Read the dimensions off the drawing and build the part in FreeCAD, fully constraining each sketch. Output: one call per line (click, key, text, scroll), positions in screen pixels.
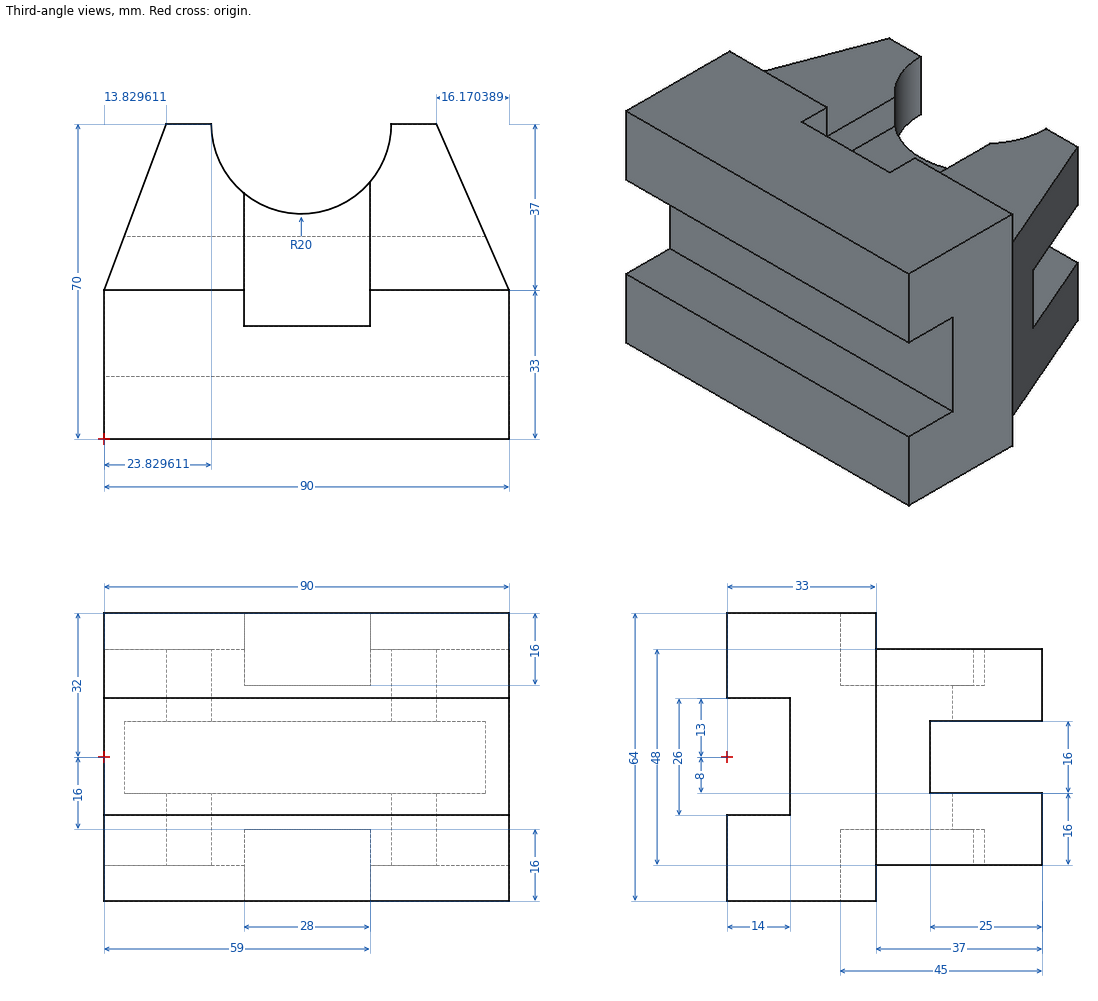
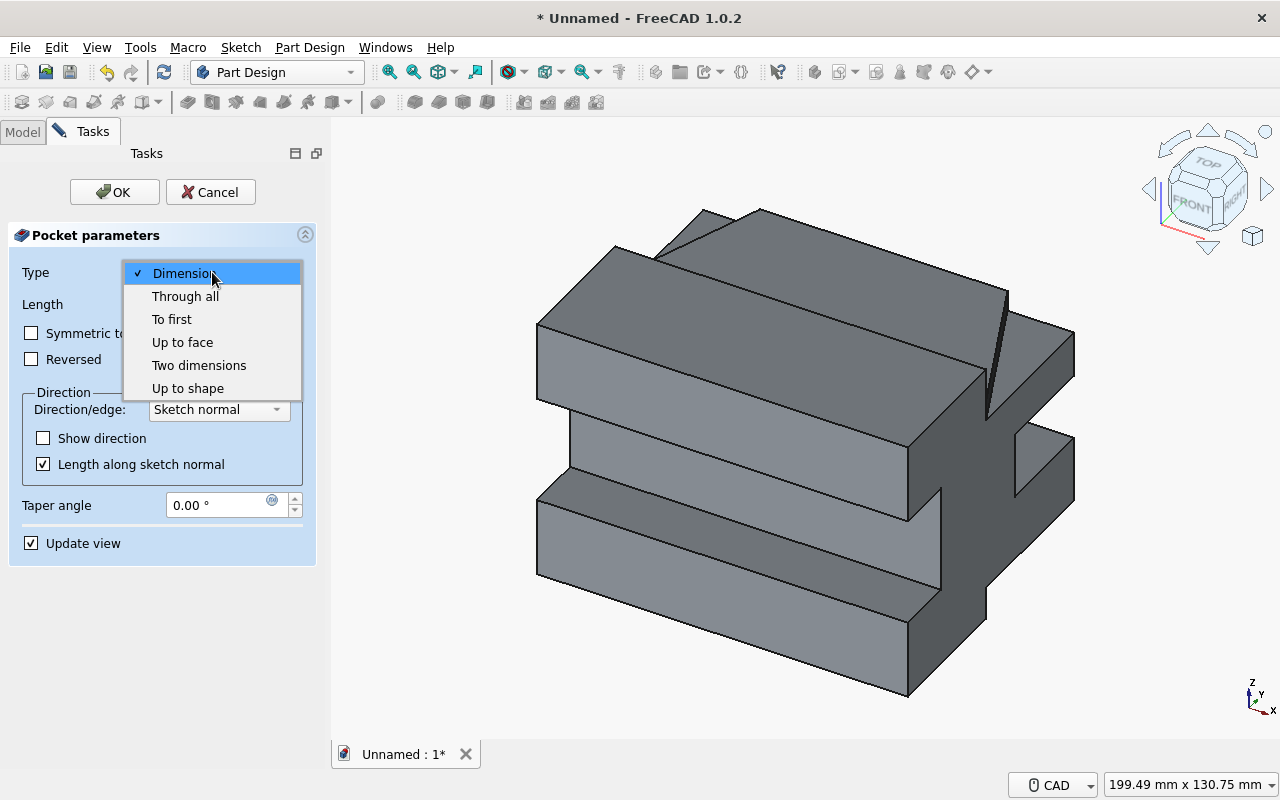
click(212, 296)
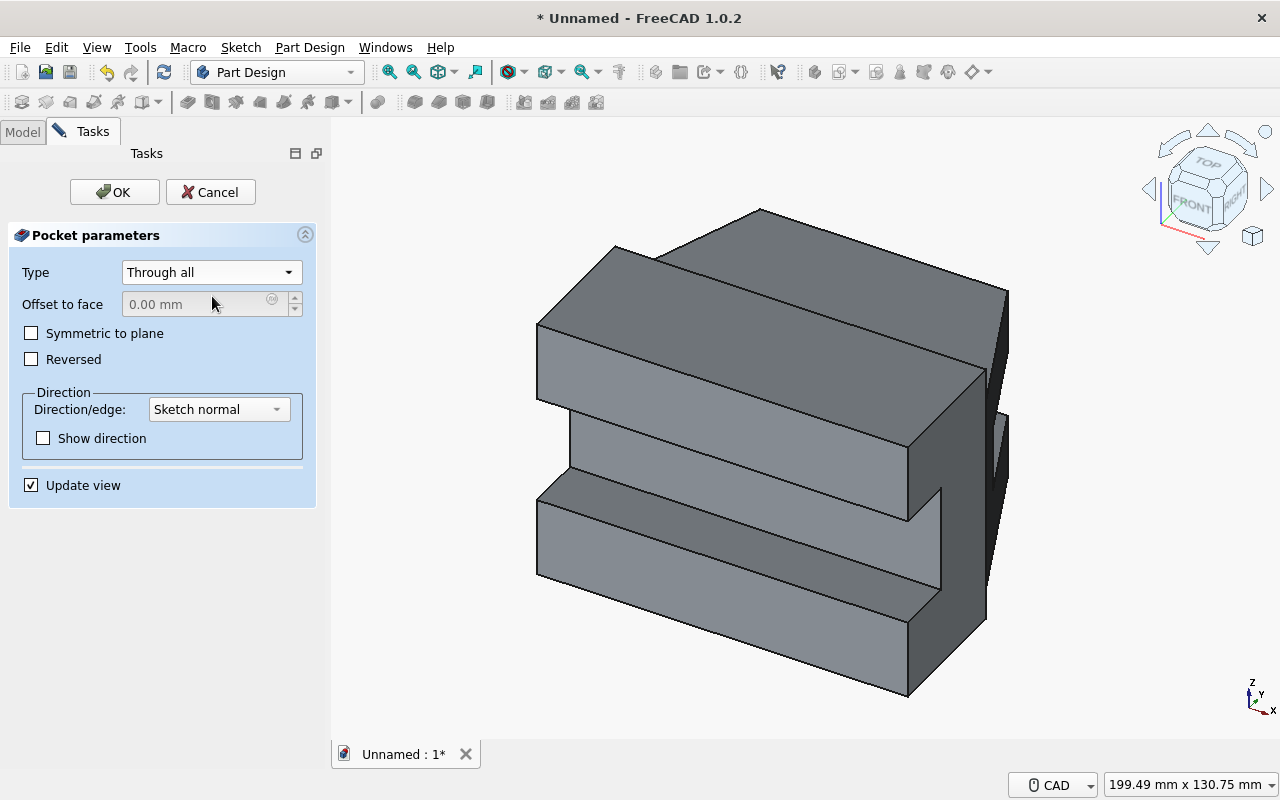
click(115, 192)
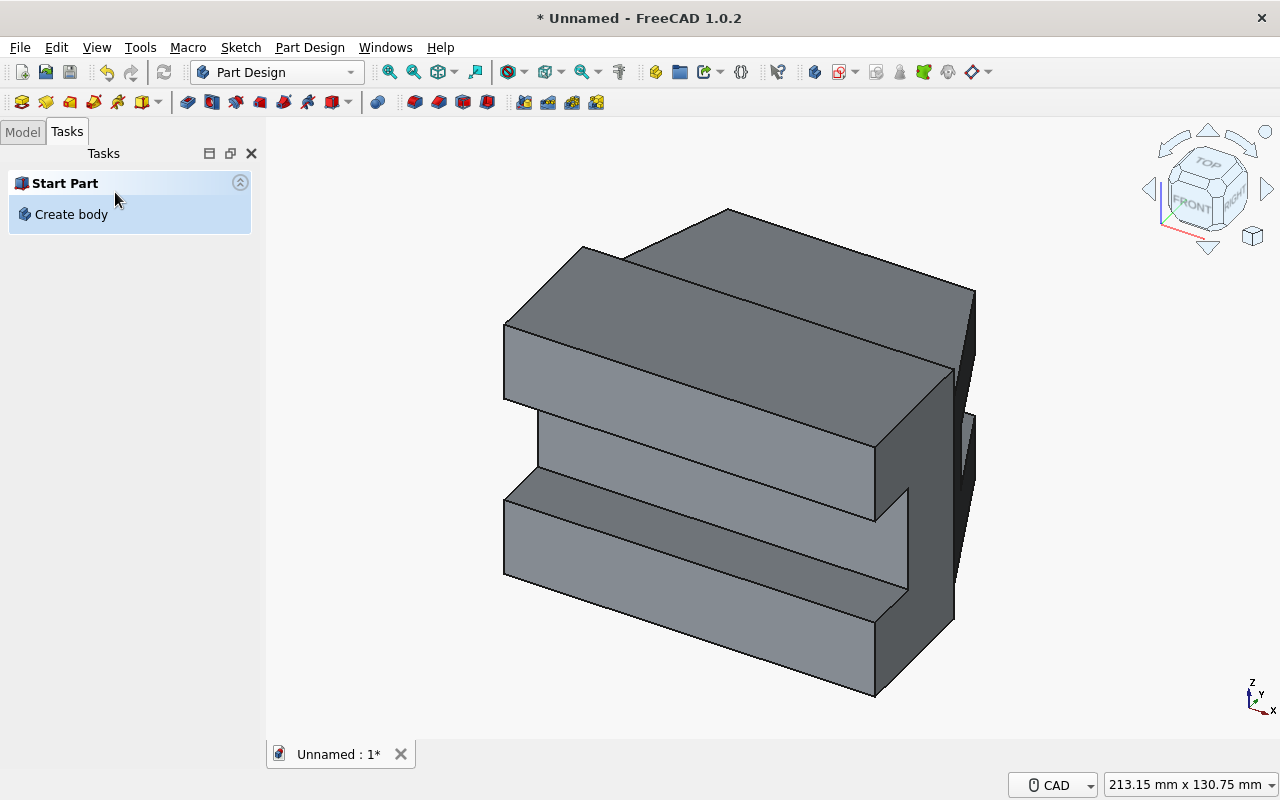
key(5)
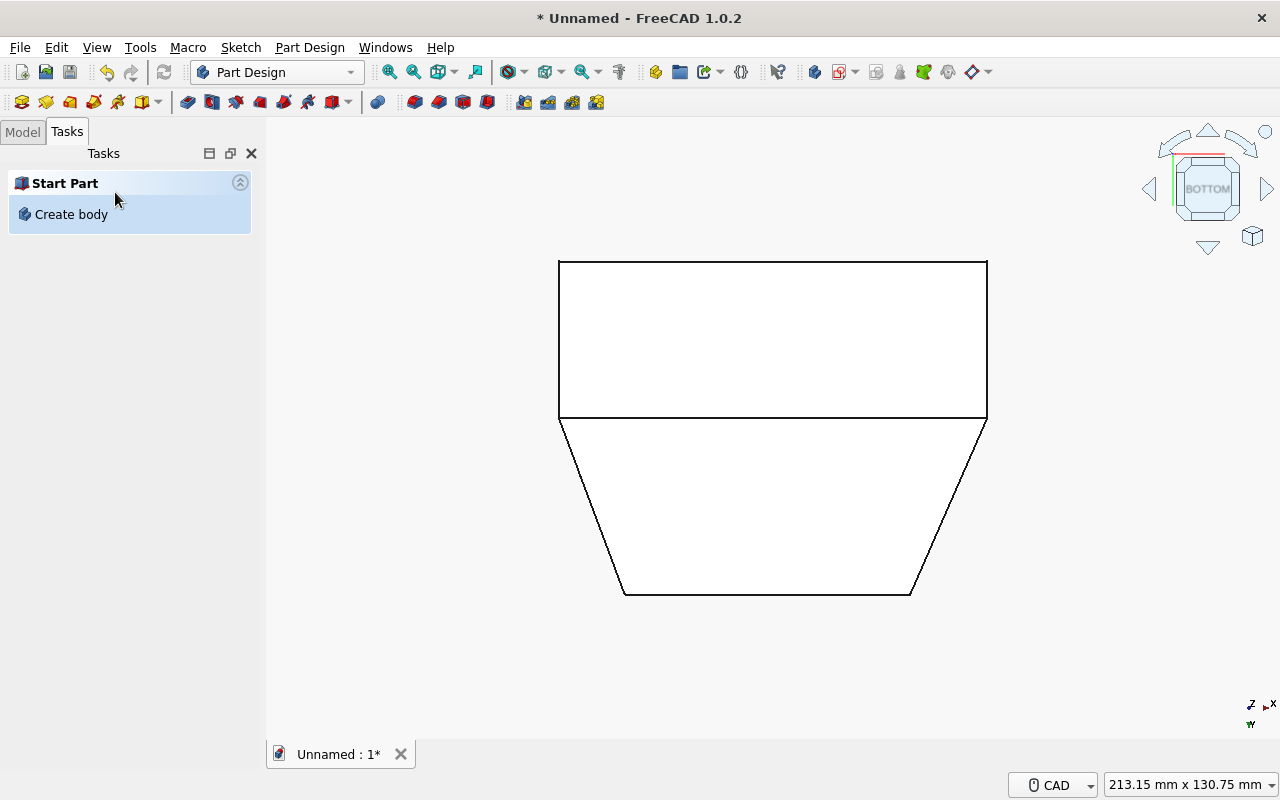
click(834, 505)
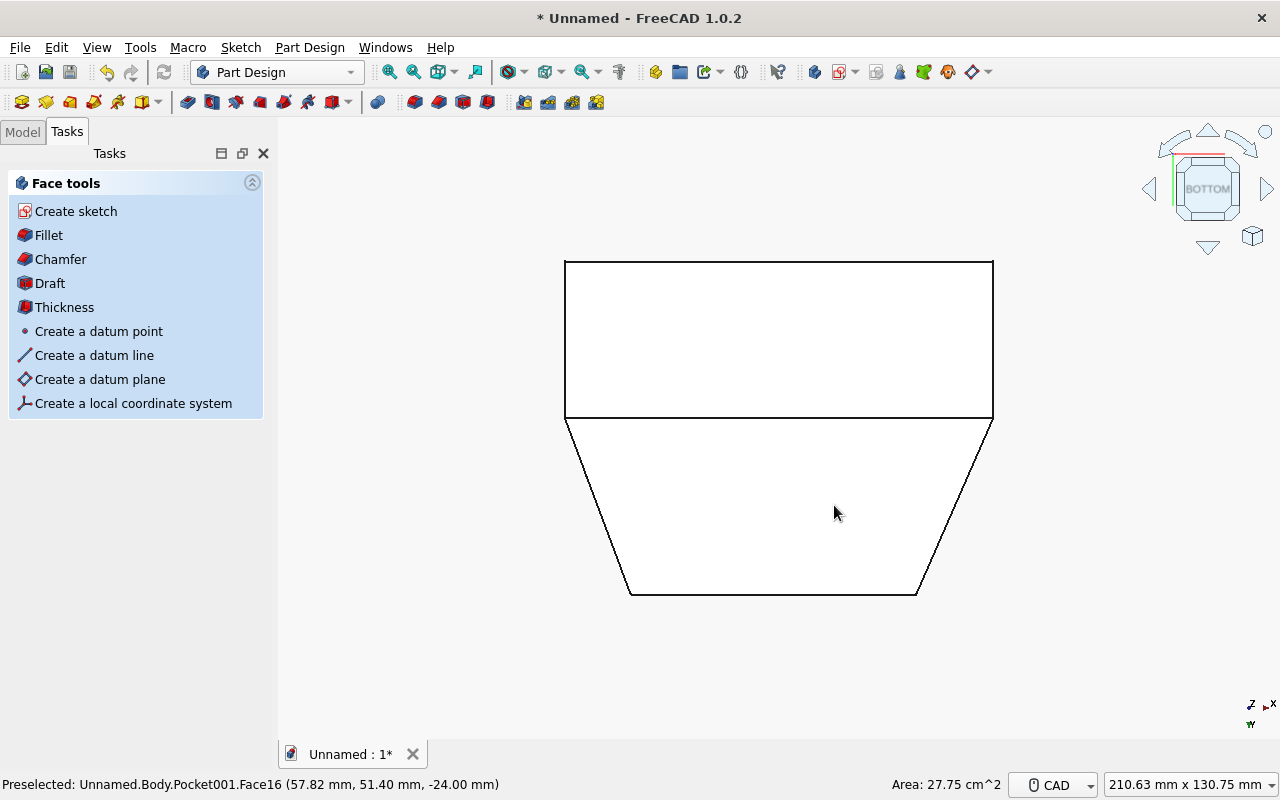
click(840, 72)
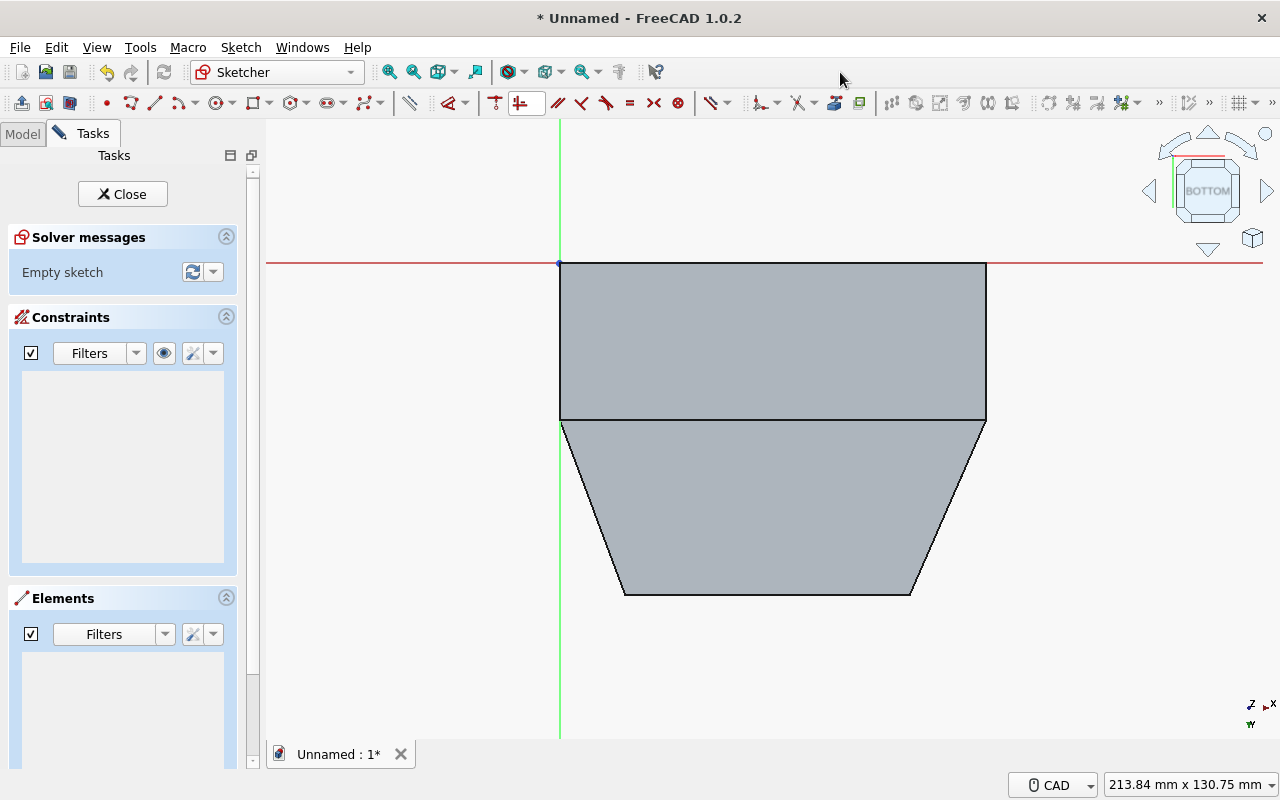
click(156, 104)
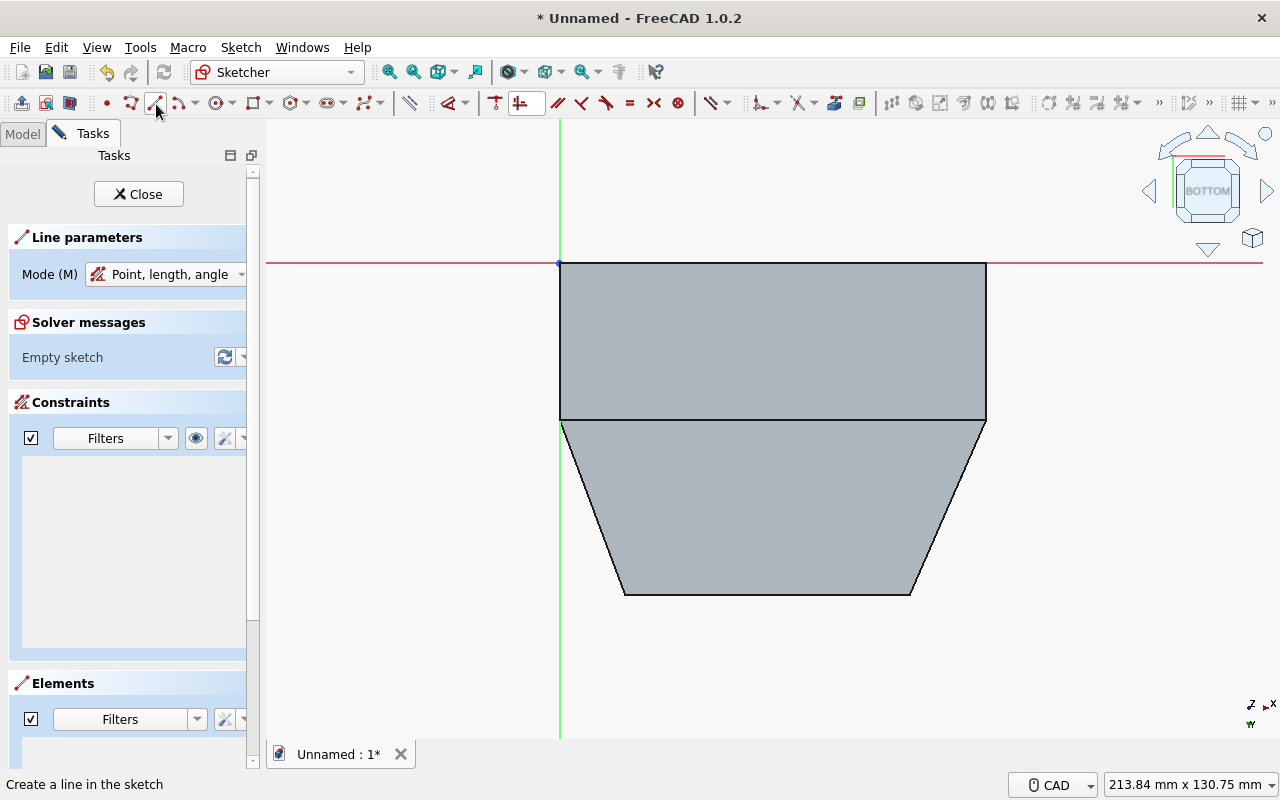
click(673, 595)
click(862, 595)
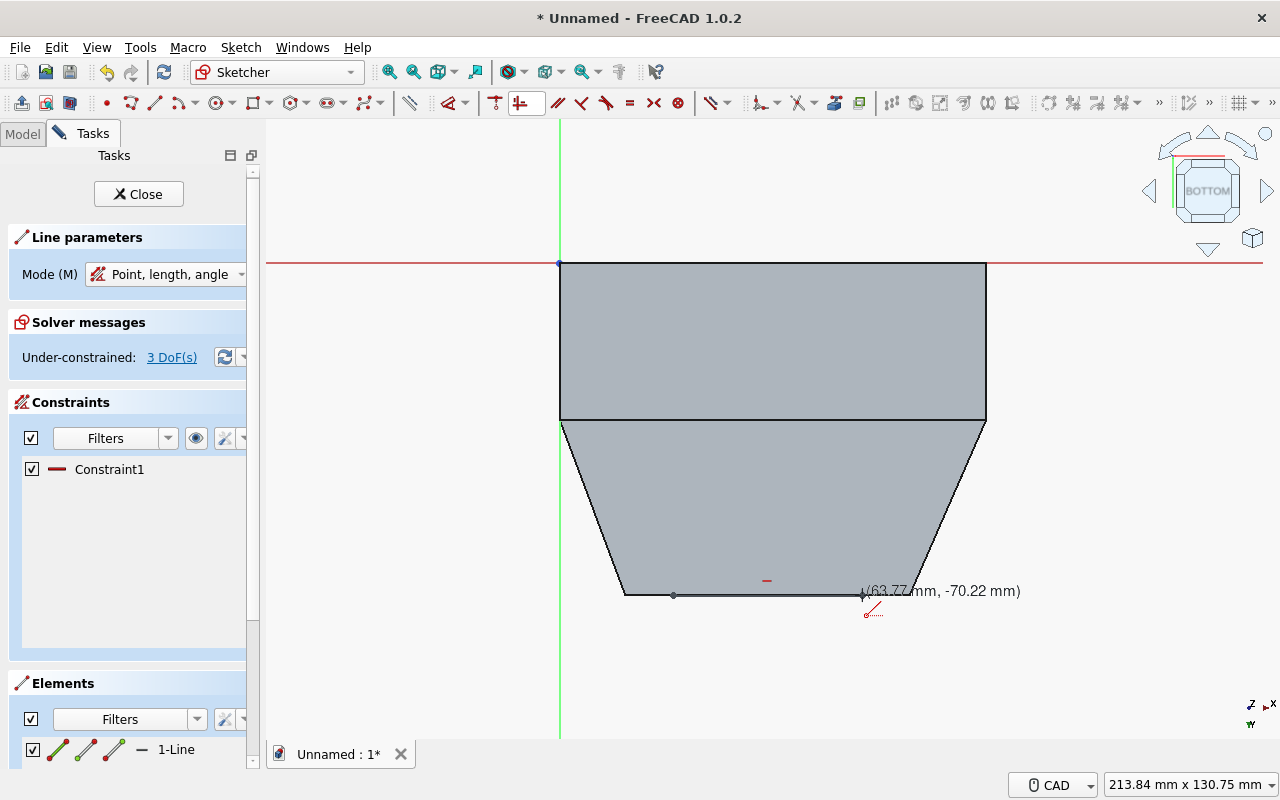
key(g)
key(3)
key(a)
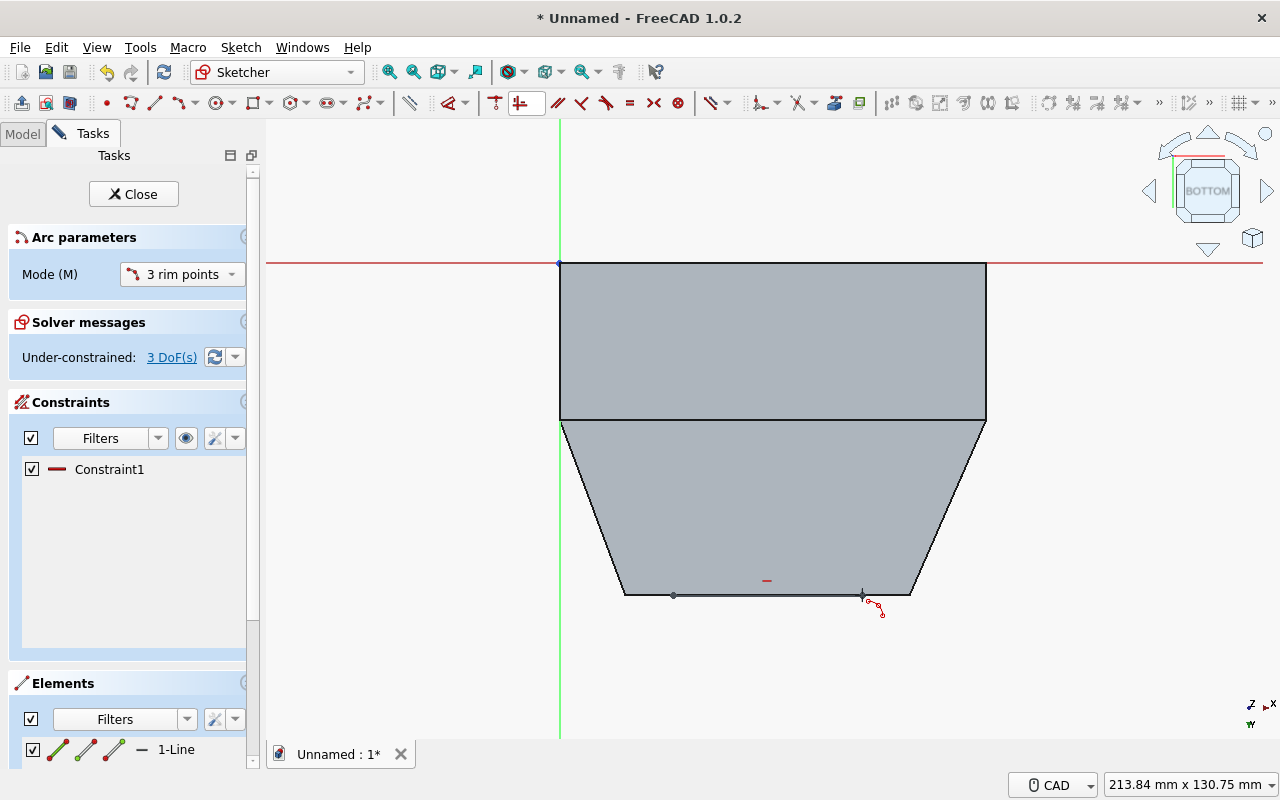
click(862, 596)
click(673, 596)
click(767, 500)
key(Escape)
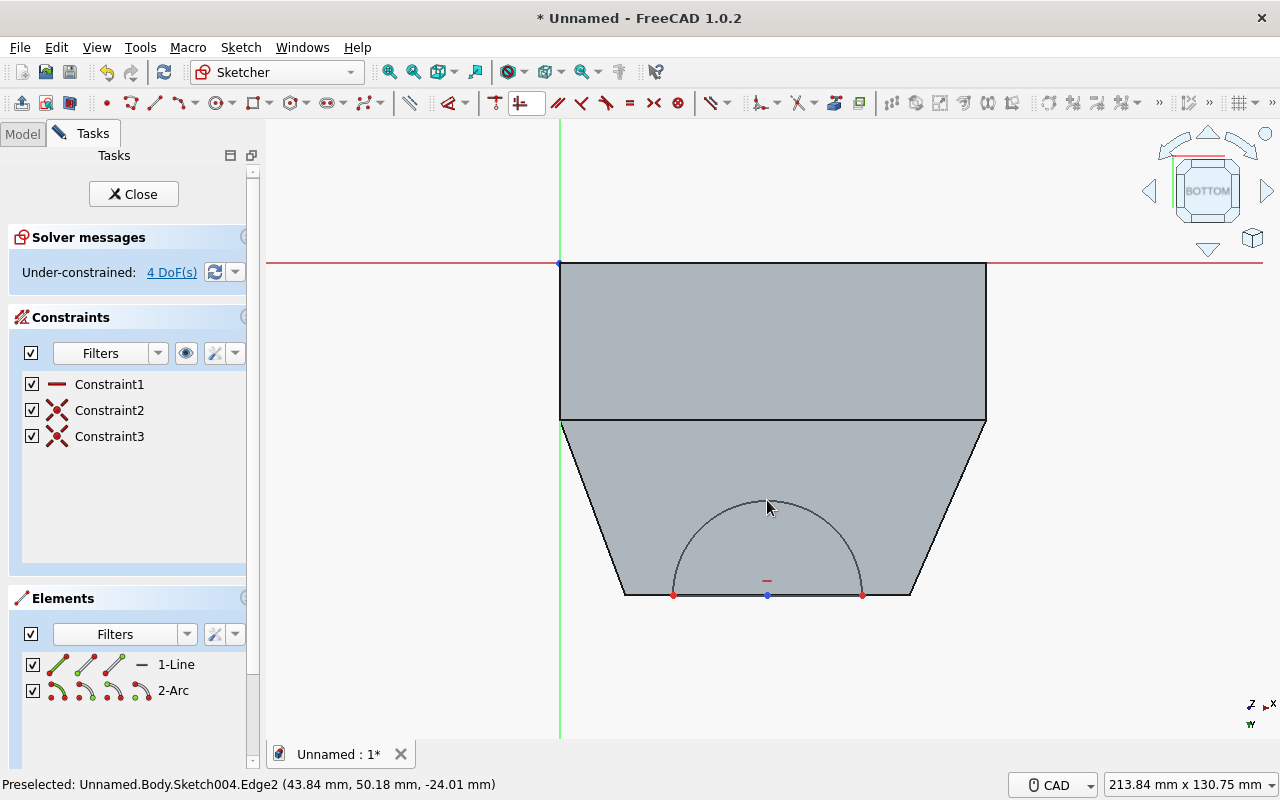
click(448, 104)